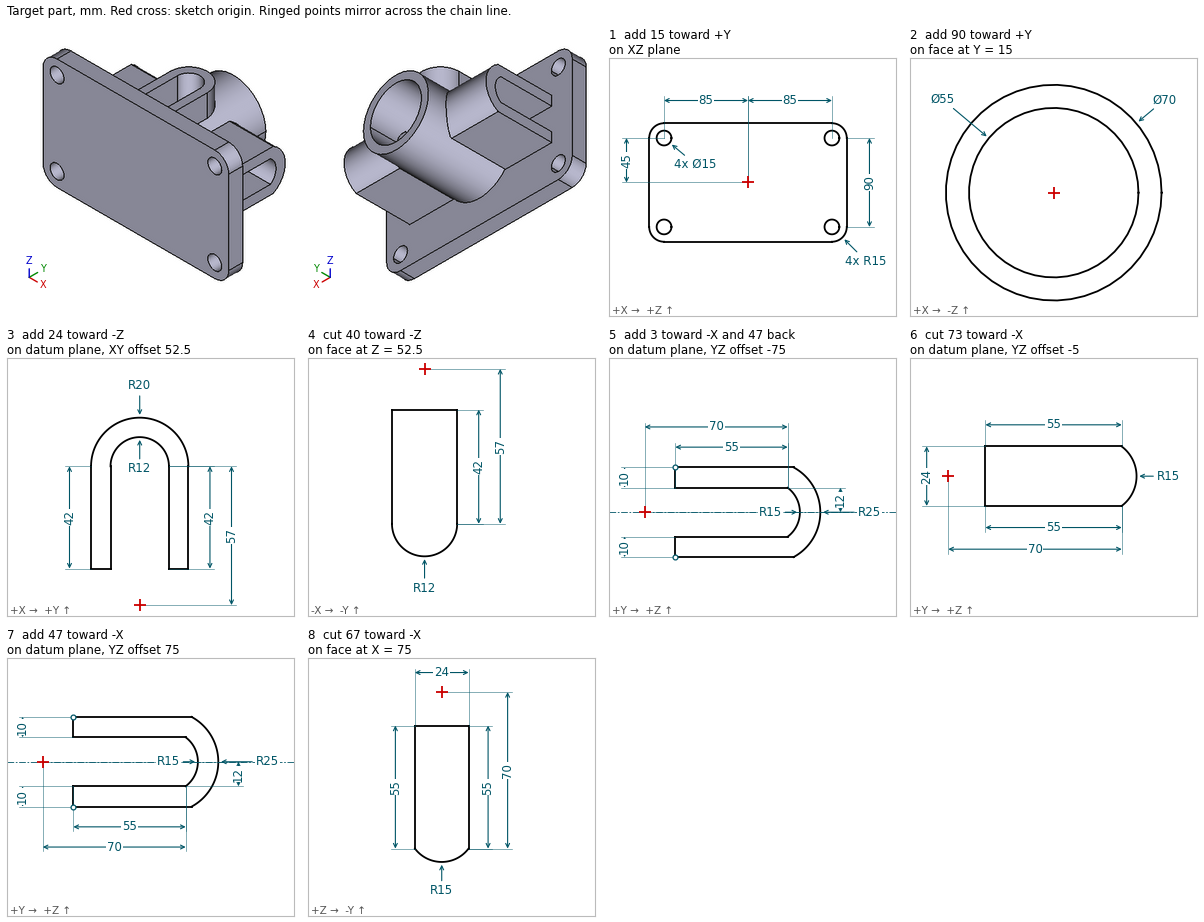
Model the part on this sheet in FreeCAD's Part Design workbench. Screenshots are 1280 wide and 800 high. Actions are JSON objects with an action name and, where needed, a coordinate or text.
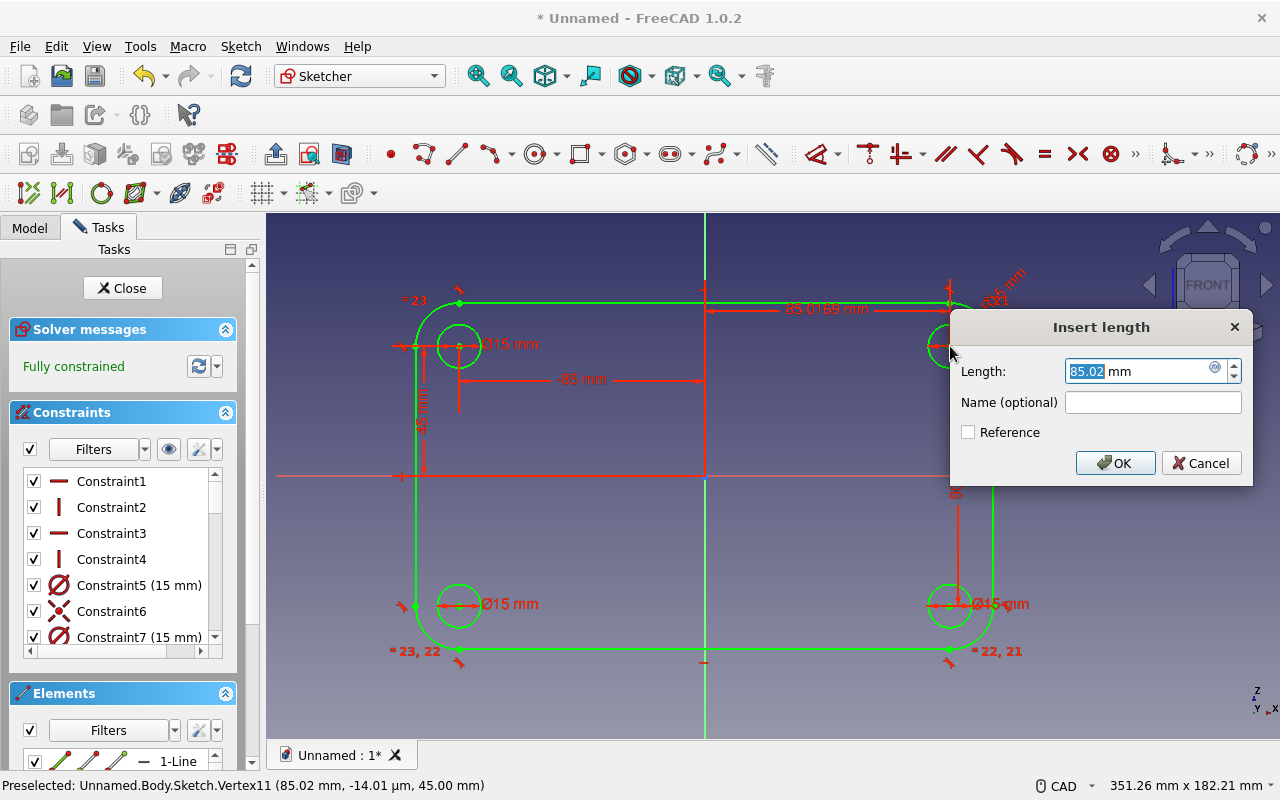
{"action": "type", "text": "85"}
{"action": "key", "text": "Return"}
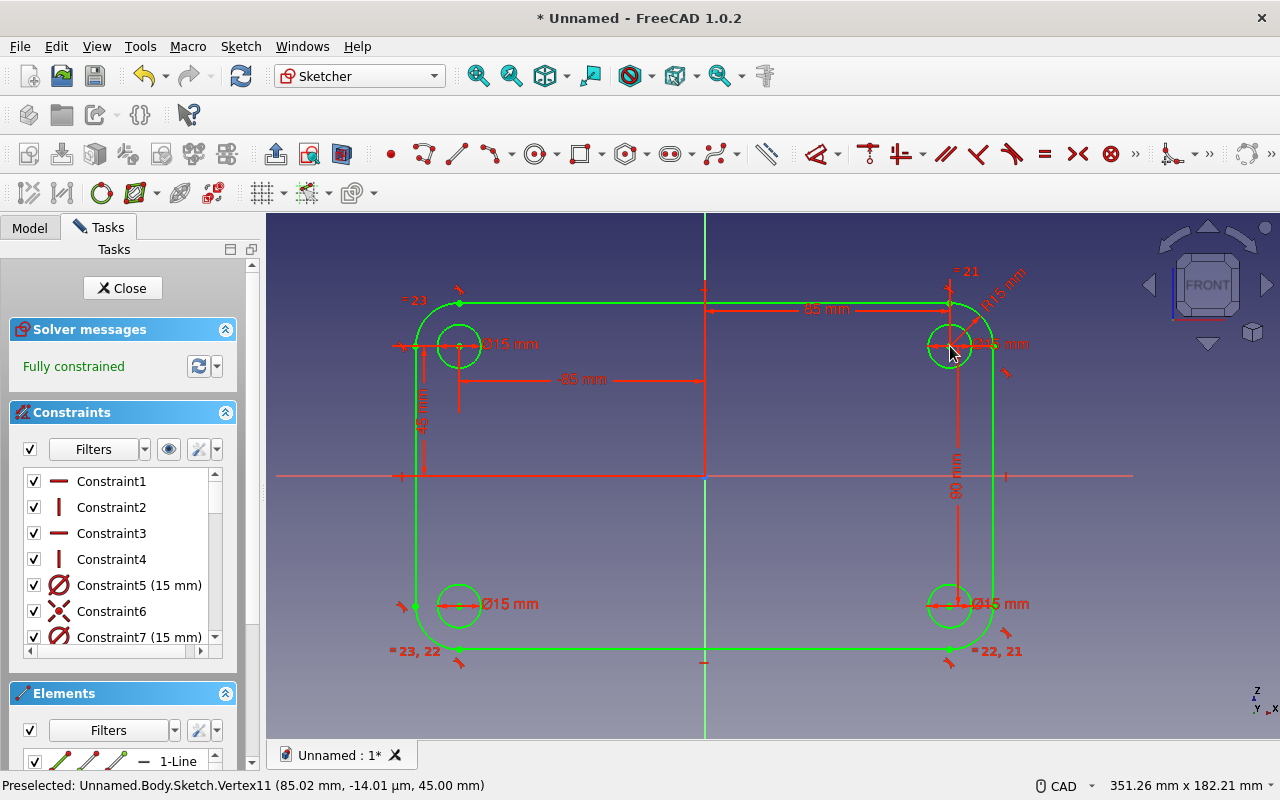
{"action": "left_click", "coordinate": [123, 288]}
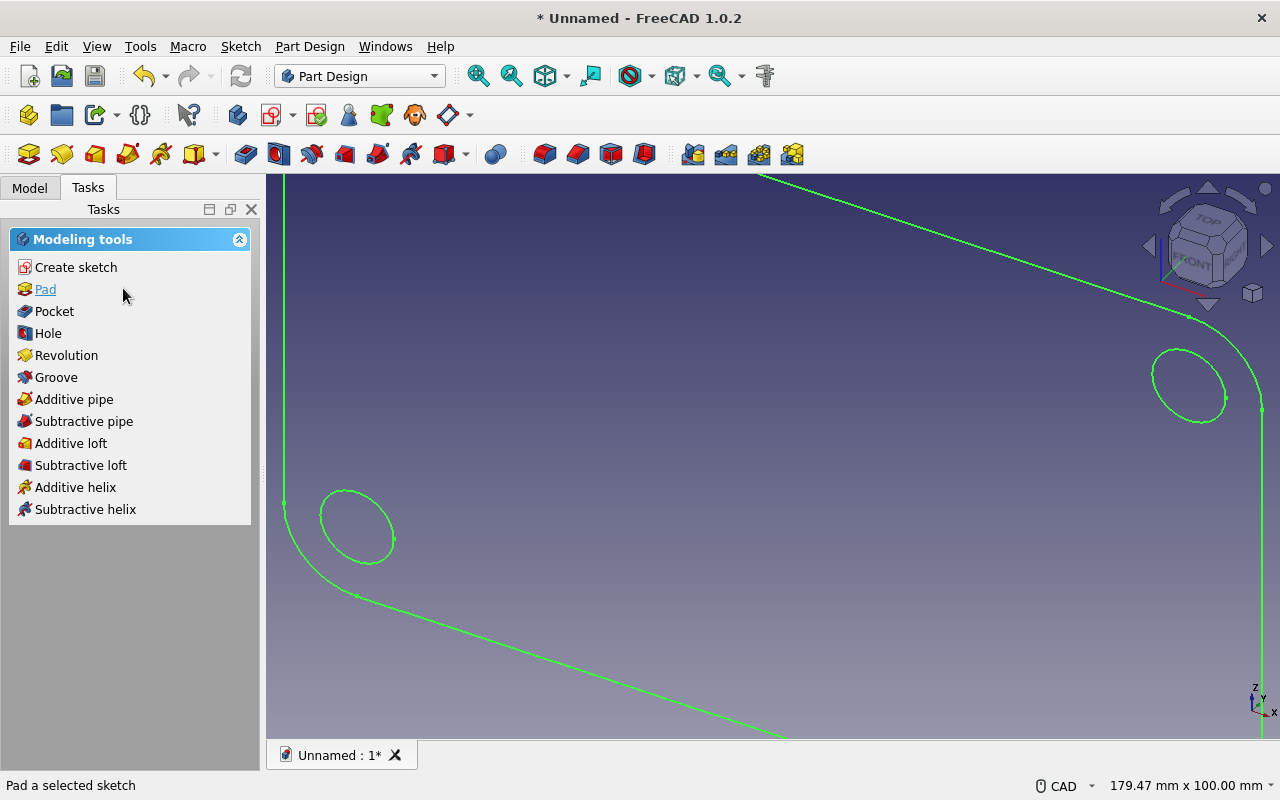
{"action": "left_click", "coordinate": [29, 154]}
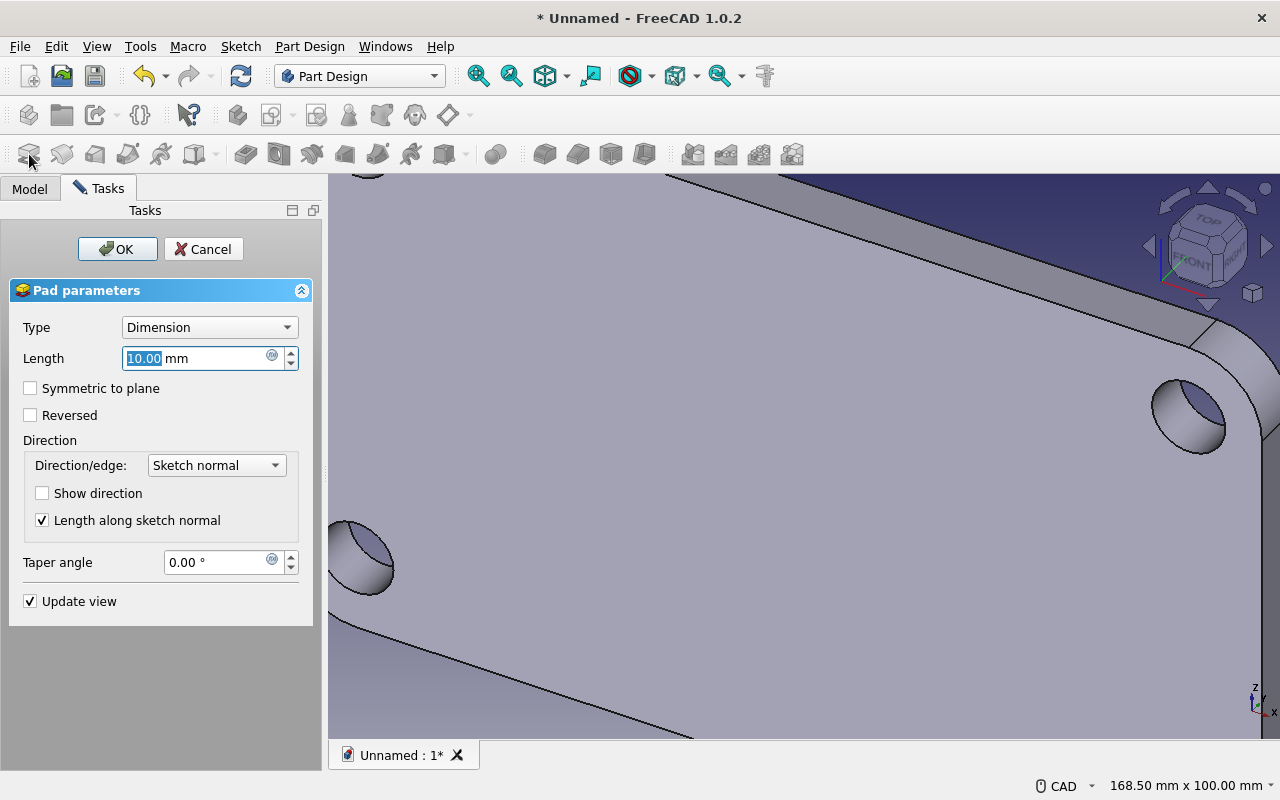
{"action": "type", "text": "15"}
{"action": "key", "text": "Tab"}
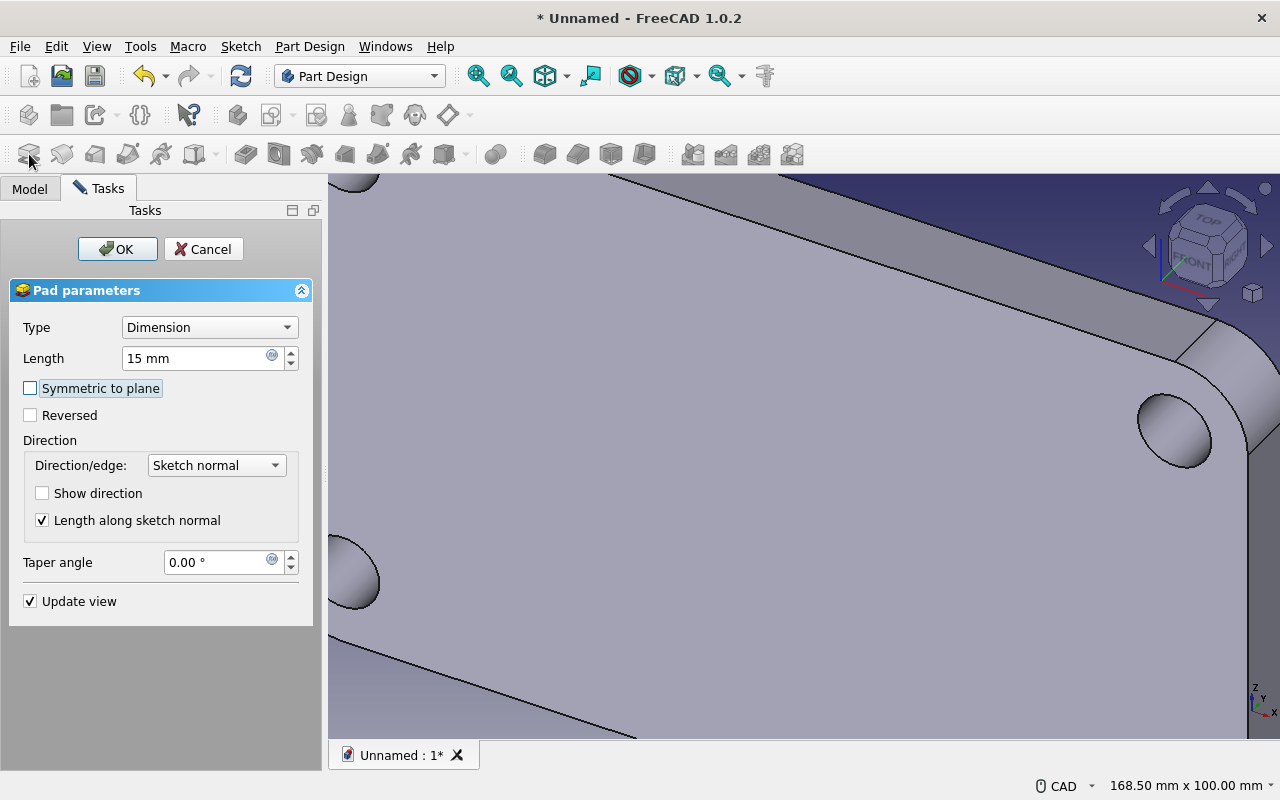
{"action": "left_click", "coordinate": [31, 415]}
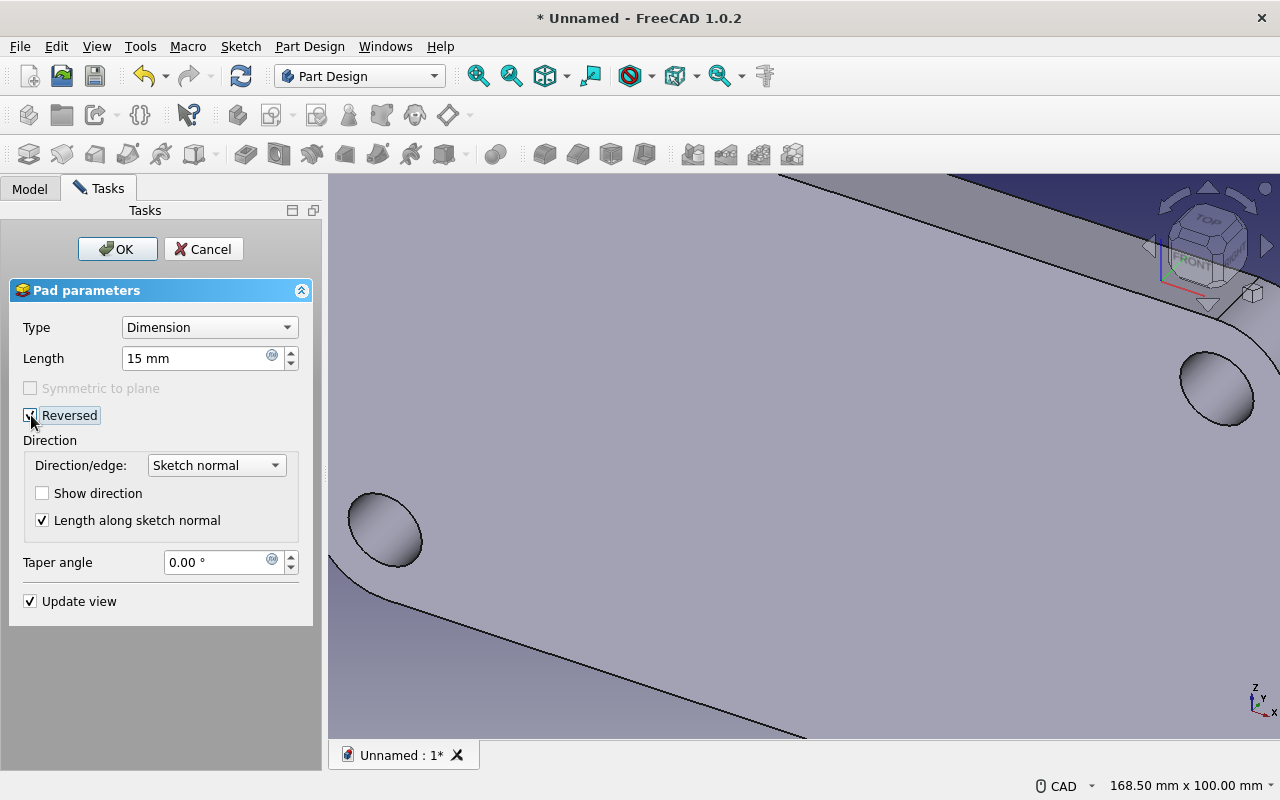
{"action": "left_click", "coordinate": [118, 249]}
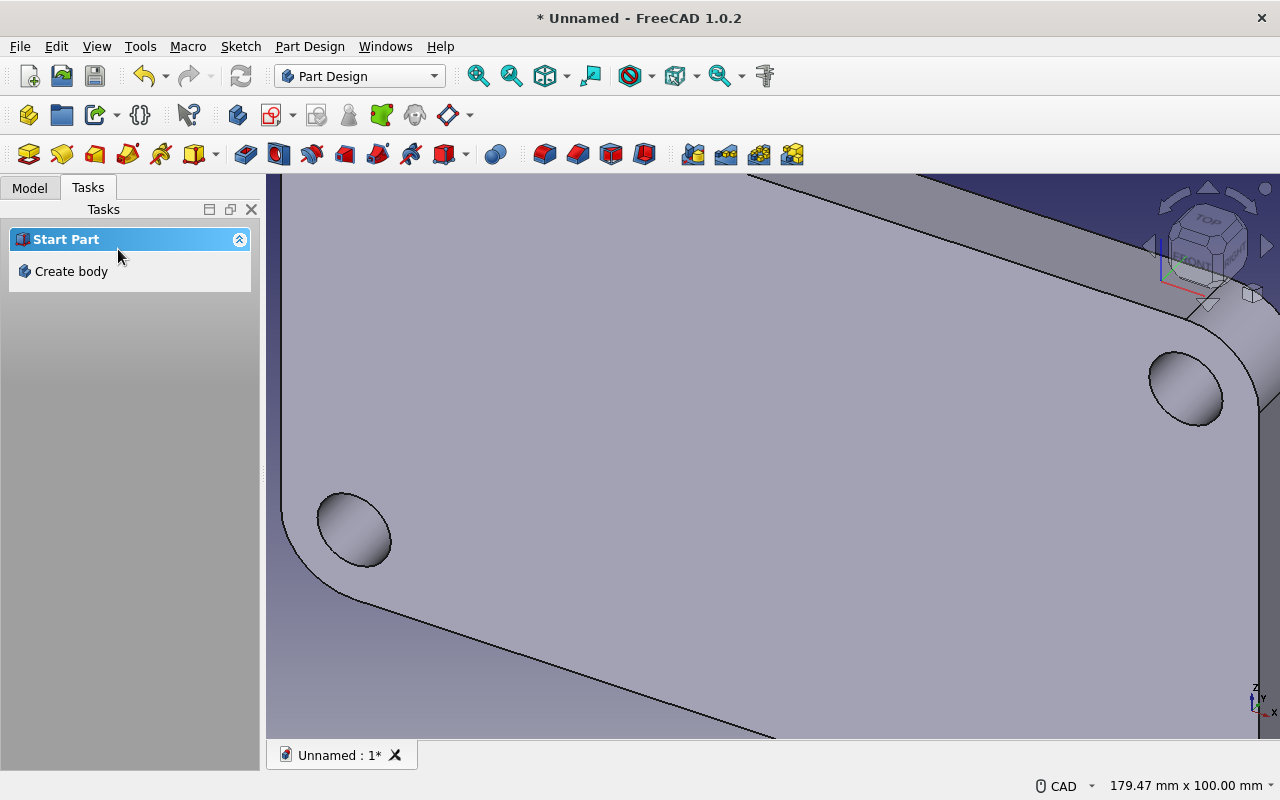
{"action": "key", "text": "v f"}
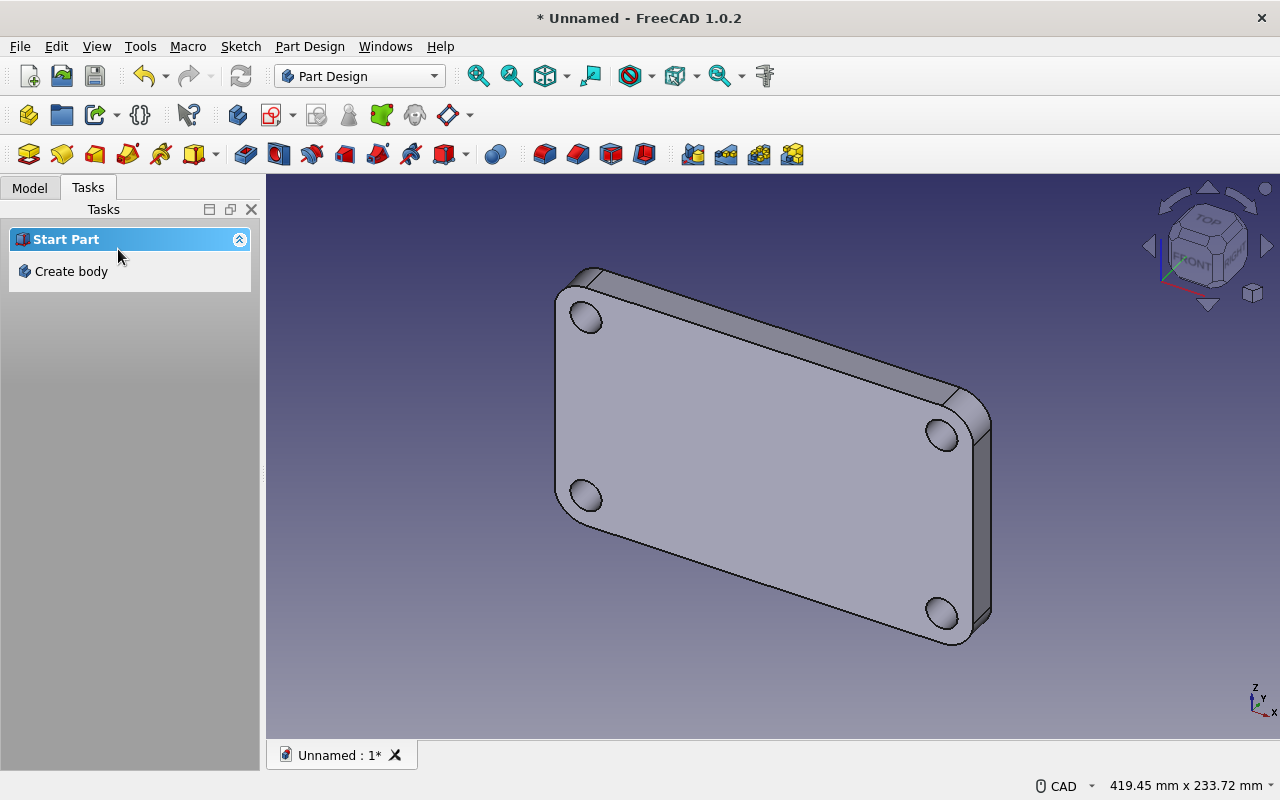
{"action": "key", "text": "4"}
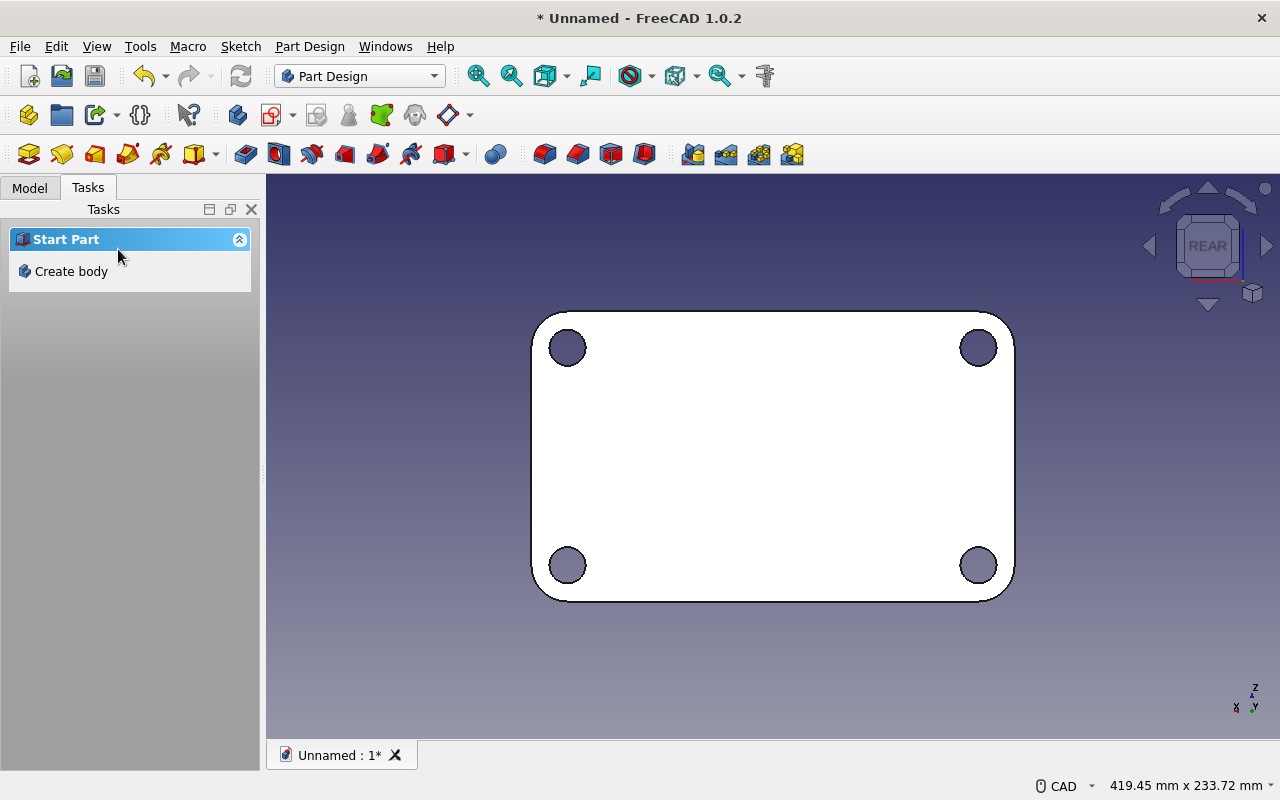
{"action": "left_click", "coordinate": [704, 456]}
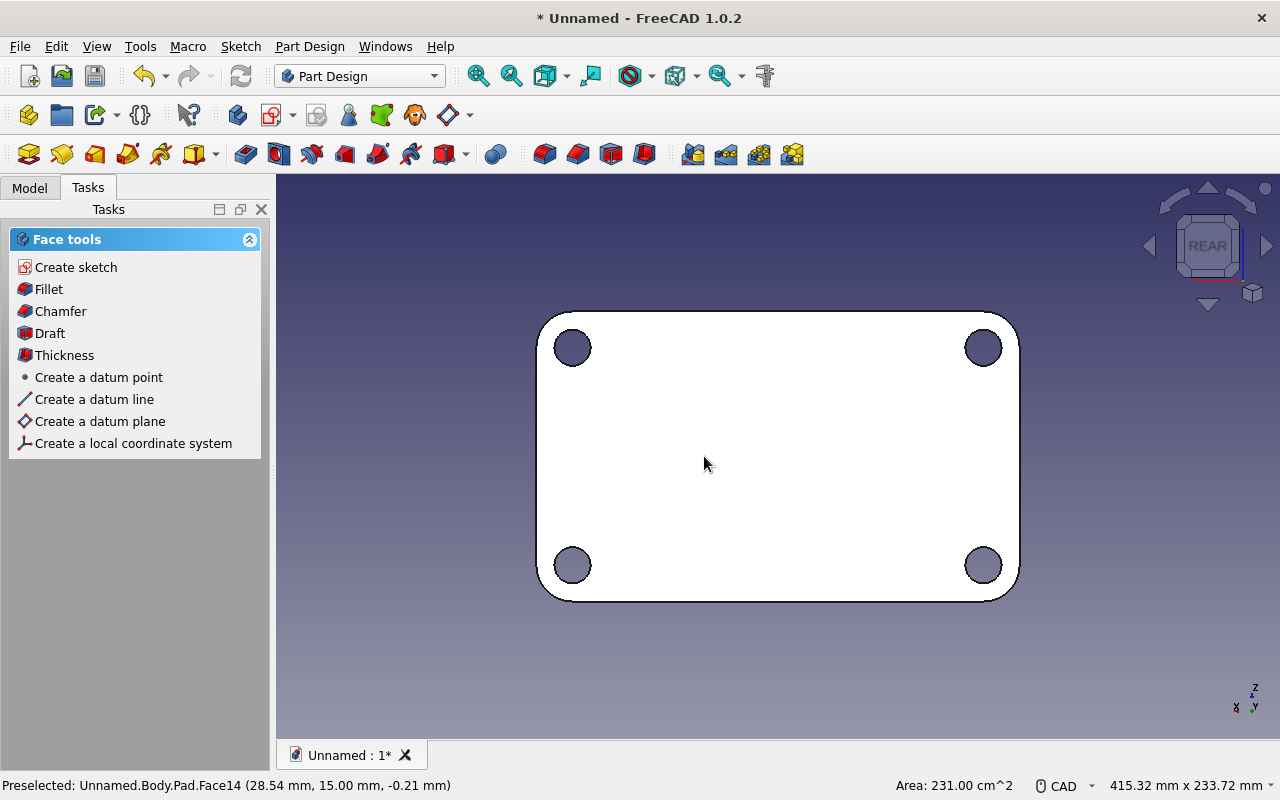
{"action": "left_click", "coordinate": [270, 116]}